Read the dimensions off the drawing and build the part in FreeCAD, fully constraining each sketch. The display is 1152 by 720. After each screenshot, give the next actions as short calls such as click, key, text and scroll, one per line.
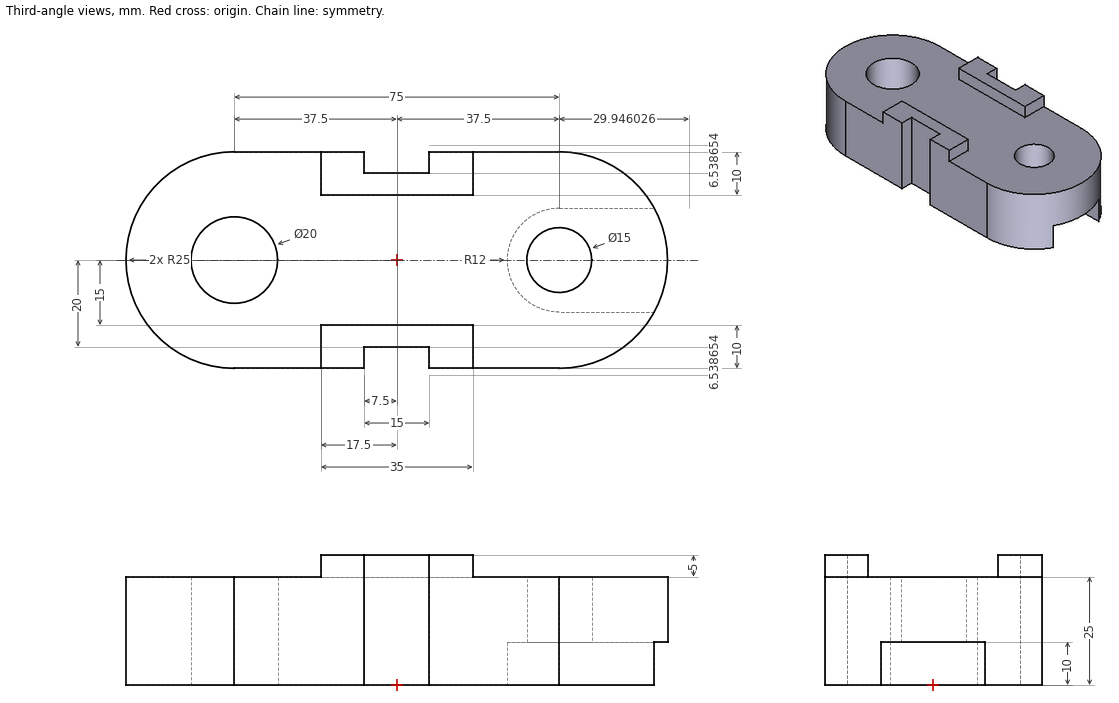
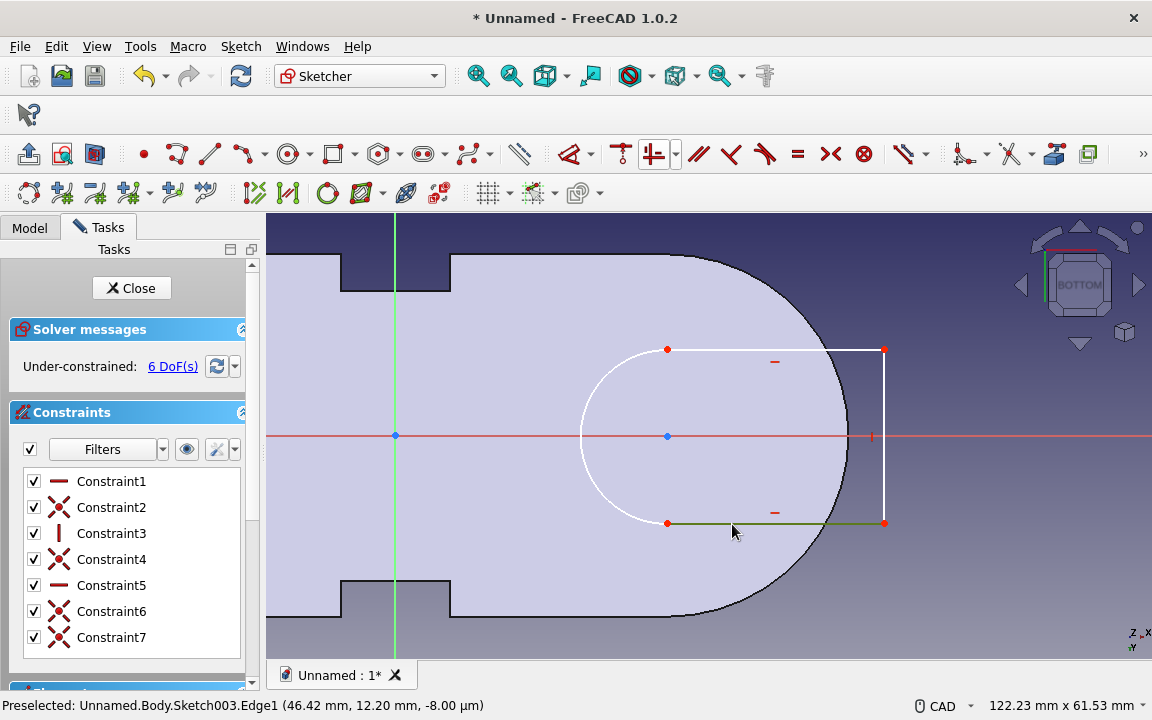
click(597, 386)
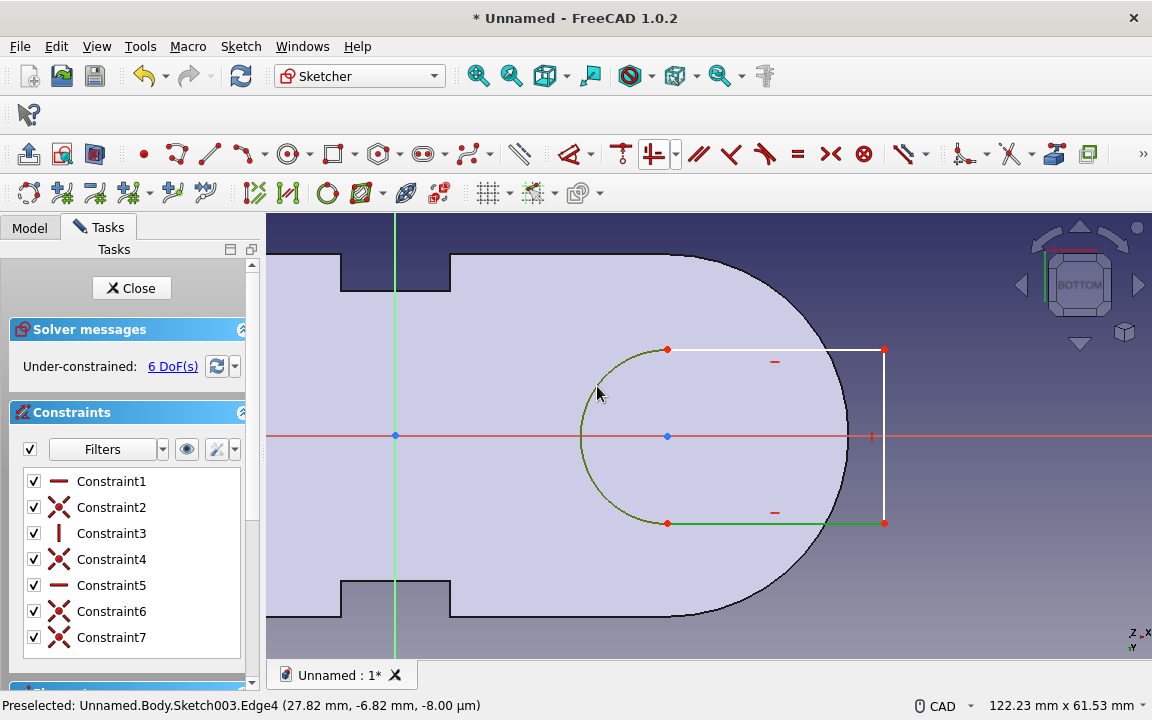
click(765, 154)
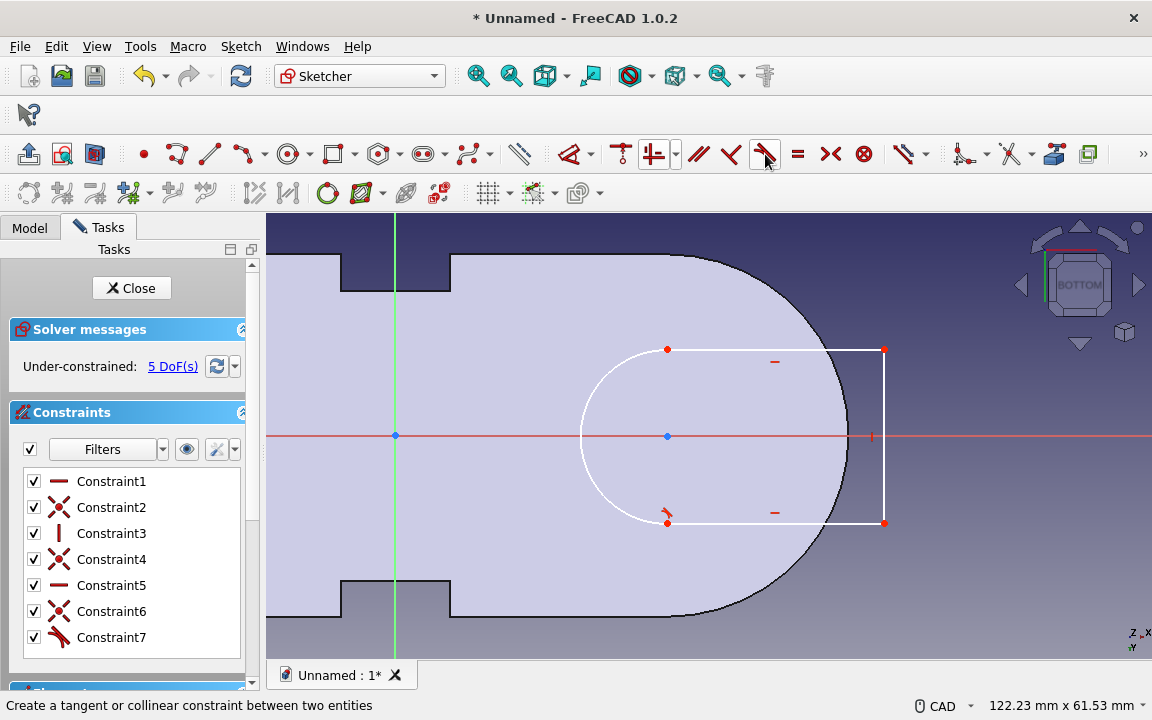
click(819, 350)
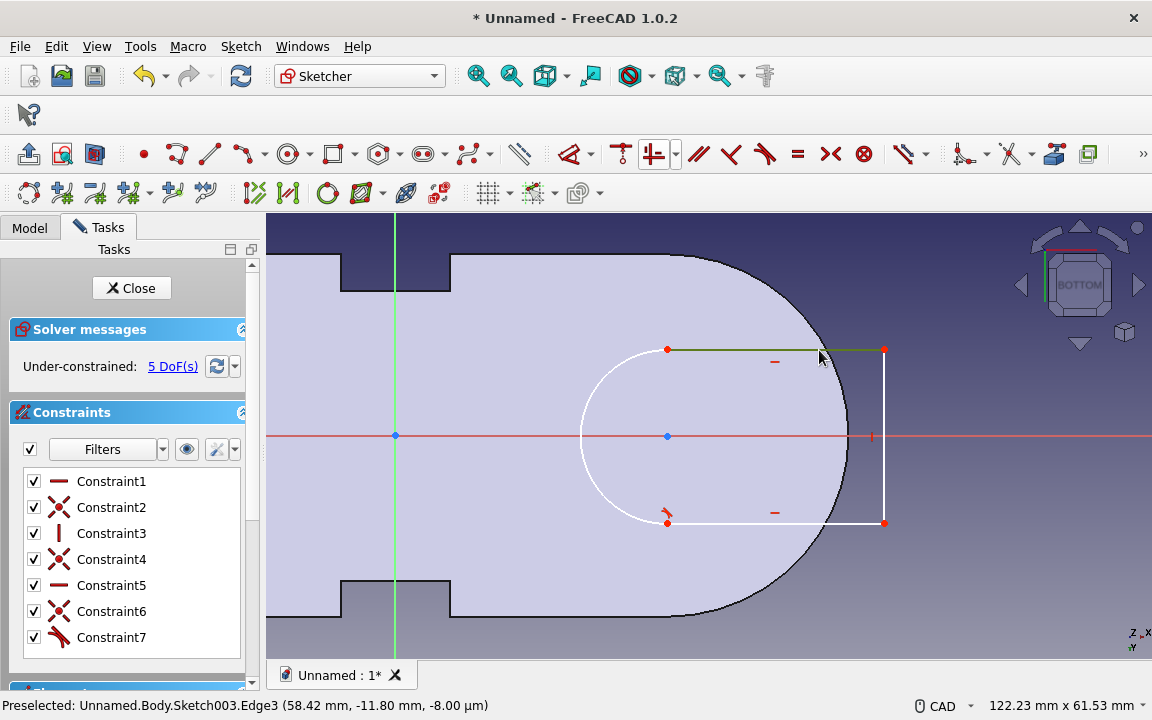
click(597, 386)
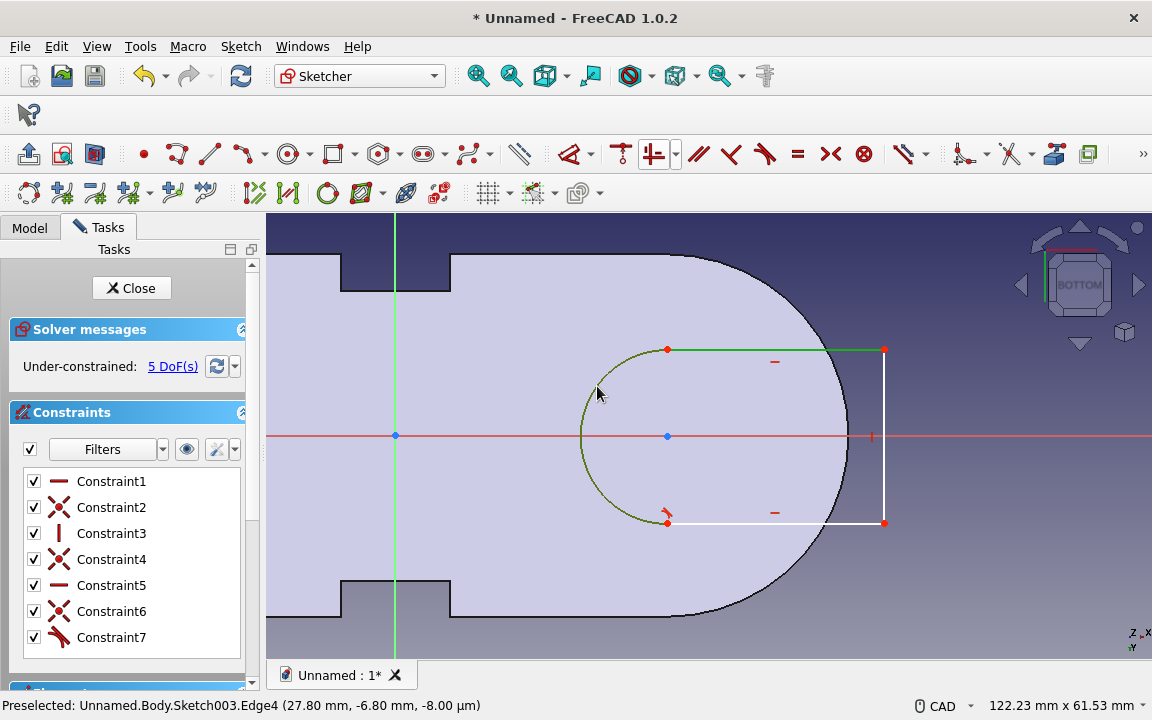
key(t)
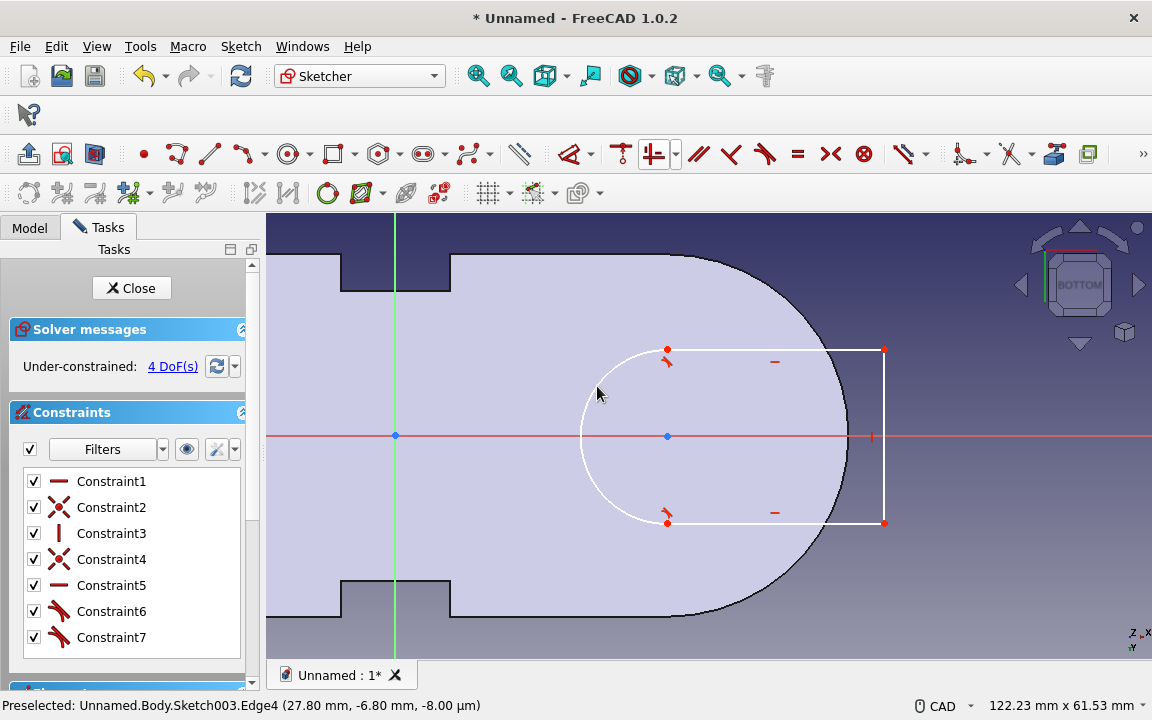
click(668, 437)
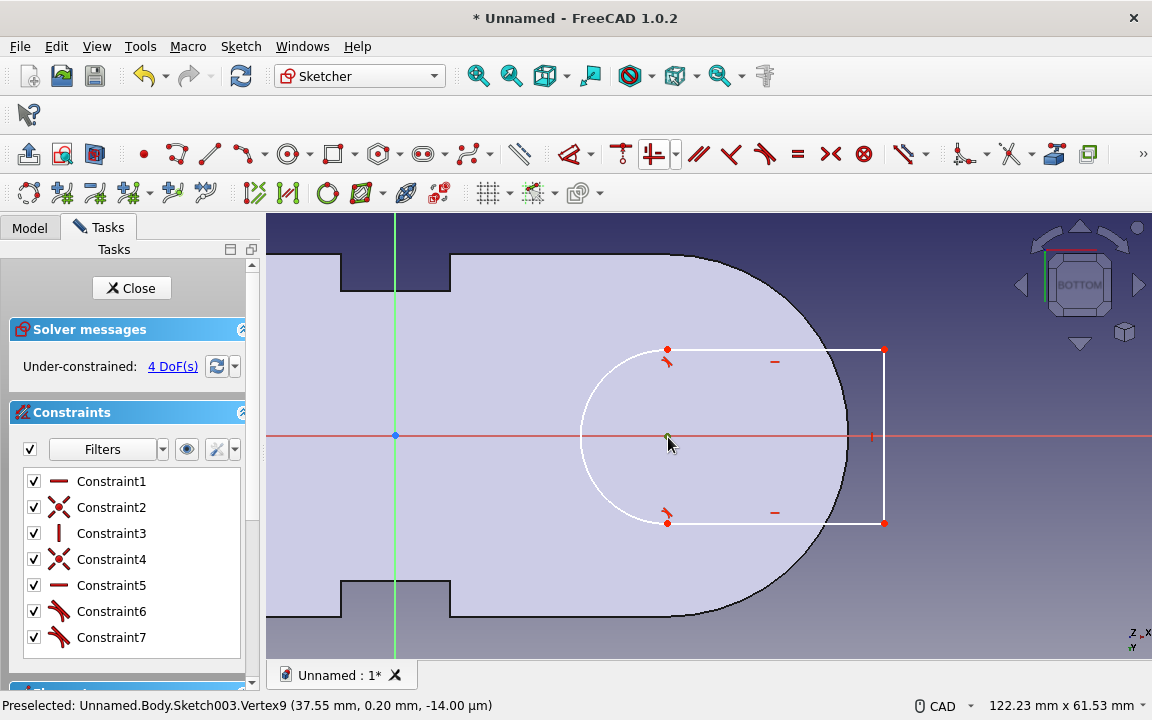
click(344, 436)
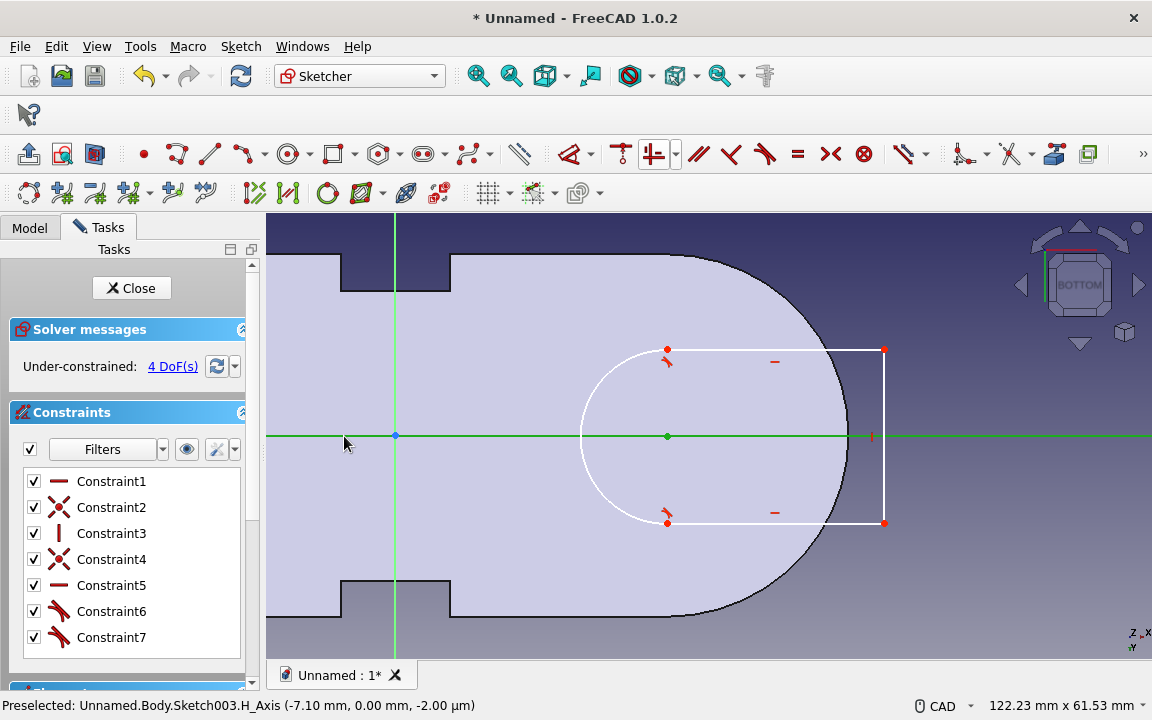
key(c)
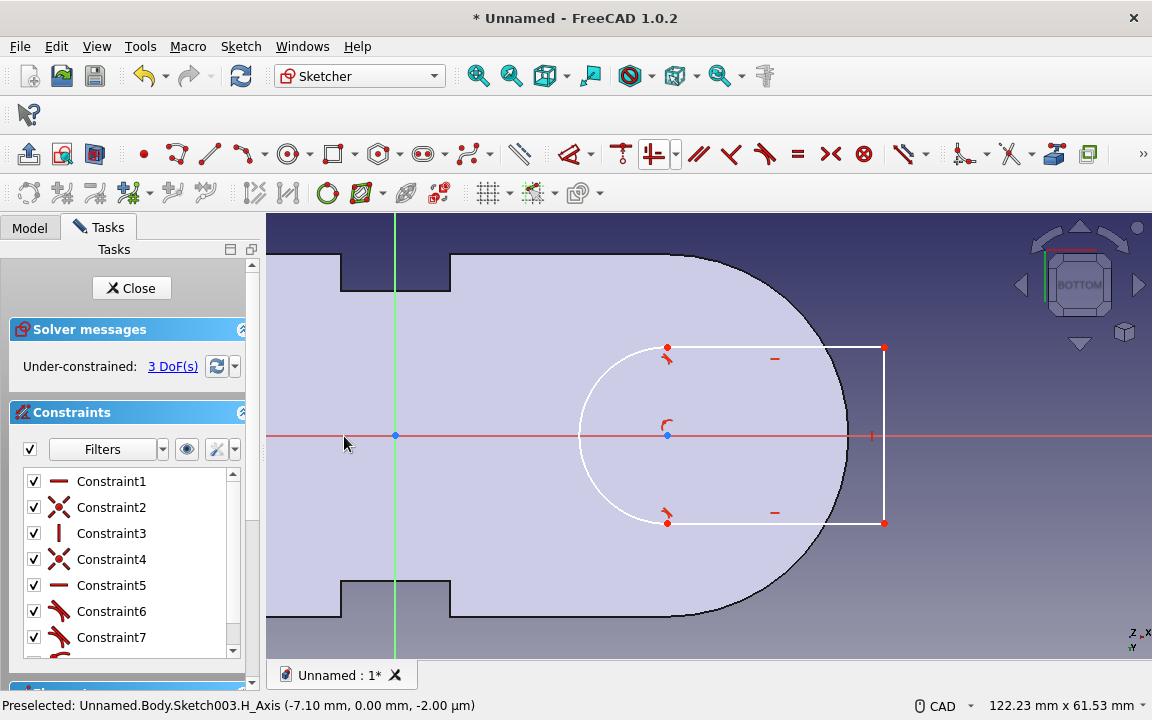
key(d)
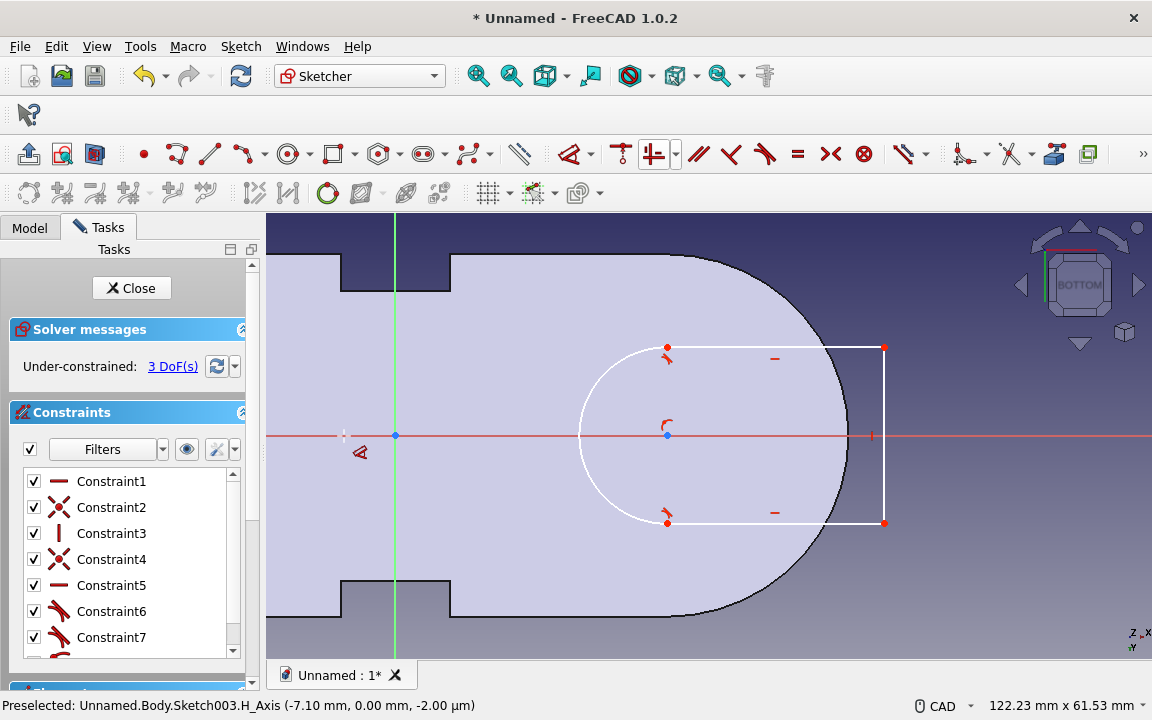
click(596, 384)
click(570, 365)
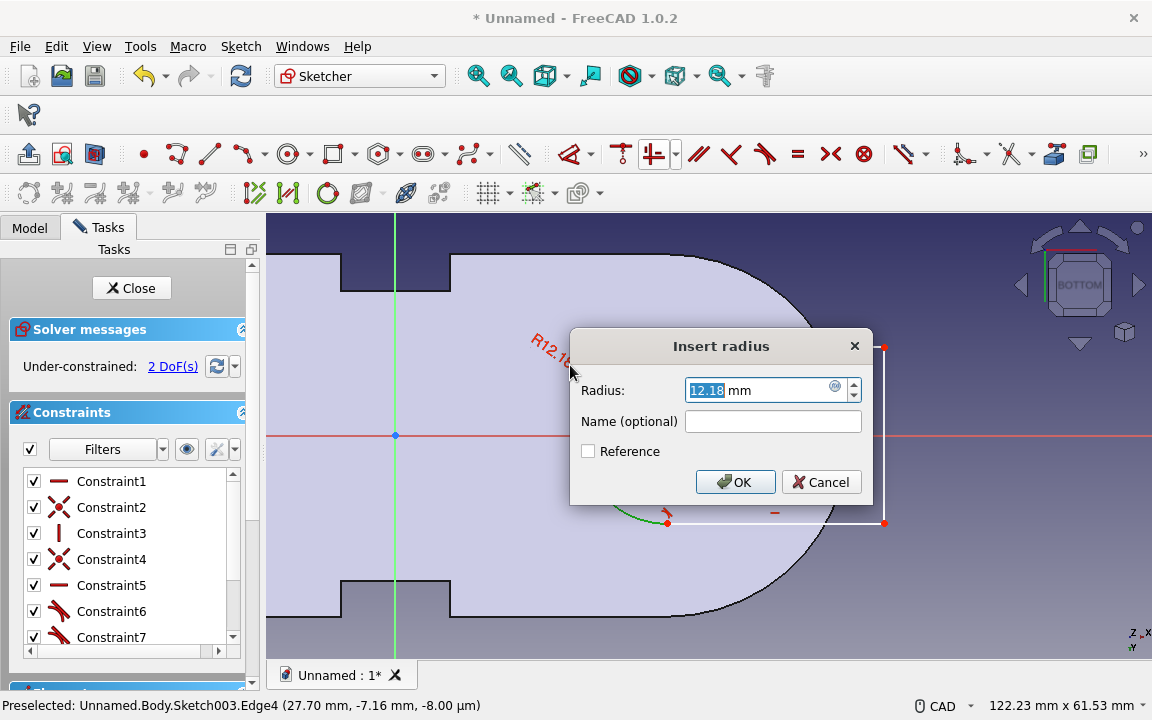
text(12)
key(Return)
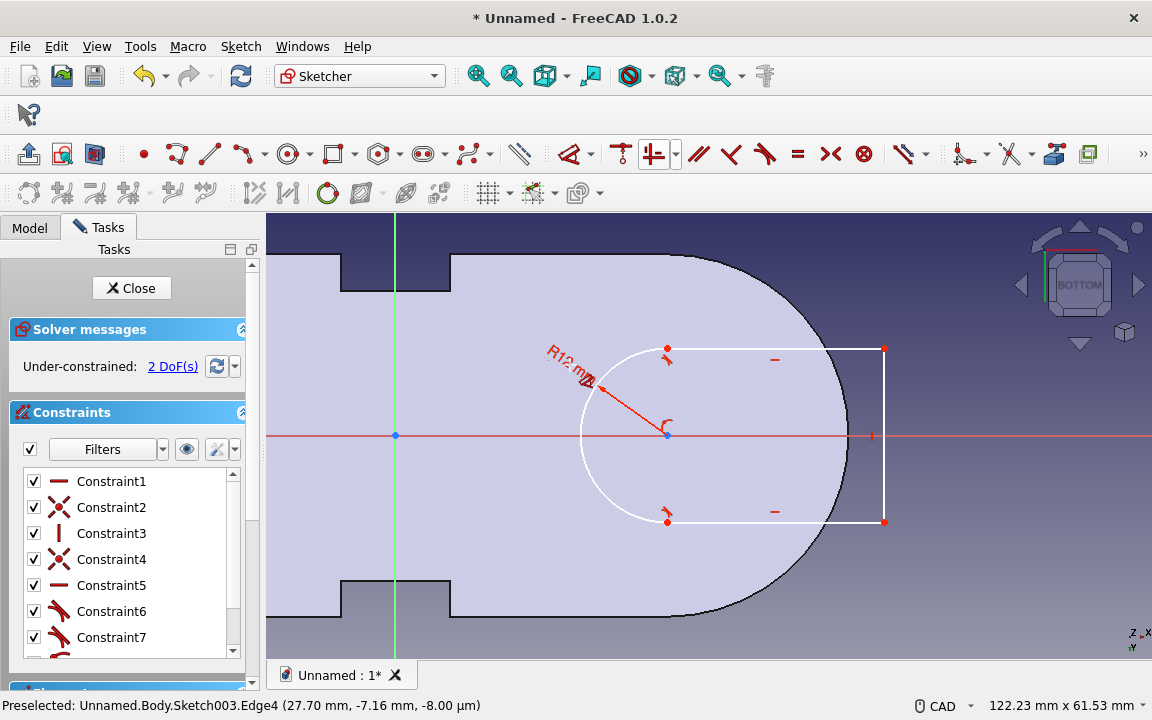
click(668, 523)
click(532, 557)